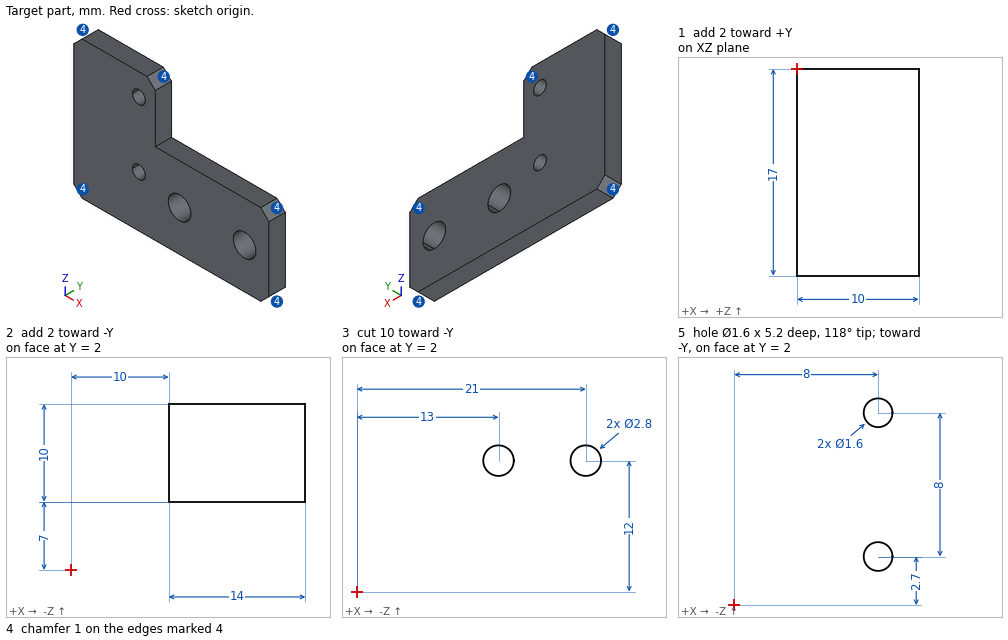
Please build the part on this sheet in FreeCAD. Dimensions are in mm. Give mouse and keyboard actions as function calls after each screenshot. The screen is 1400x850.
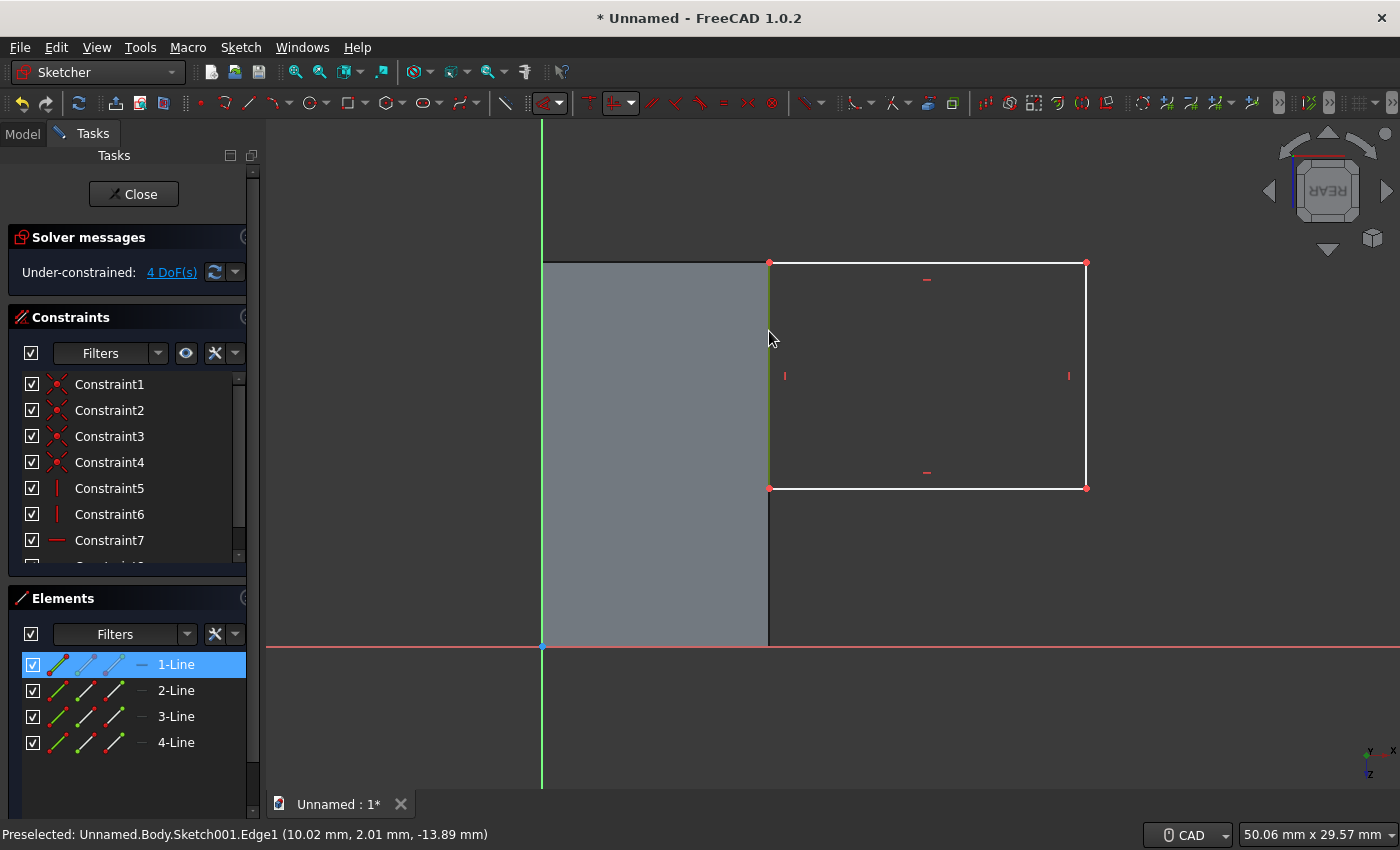
key(i)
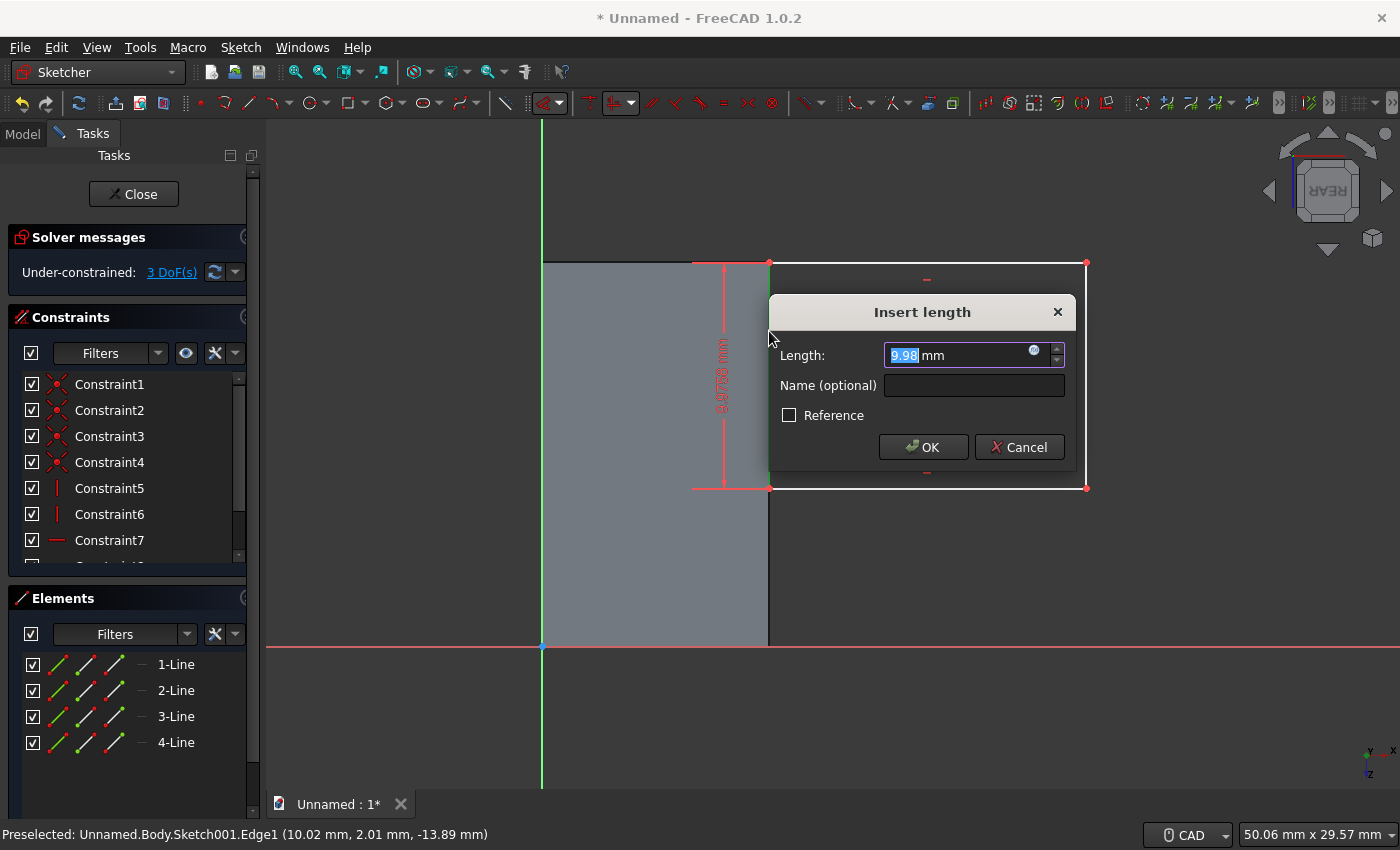
text(10)
key(Return)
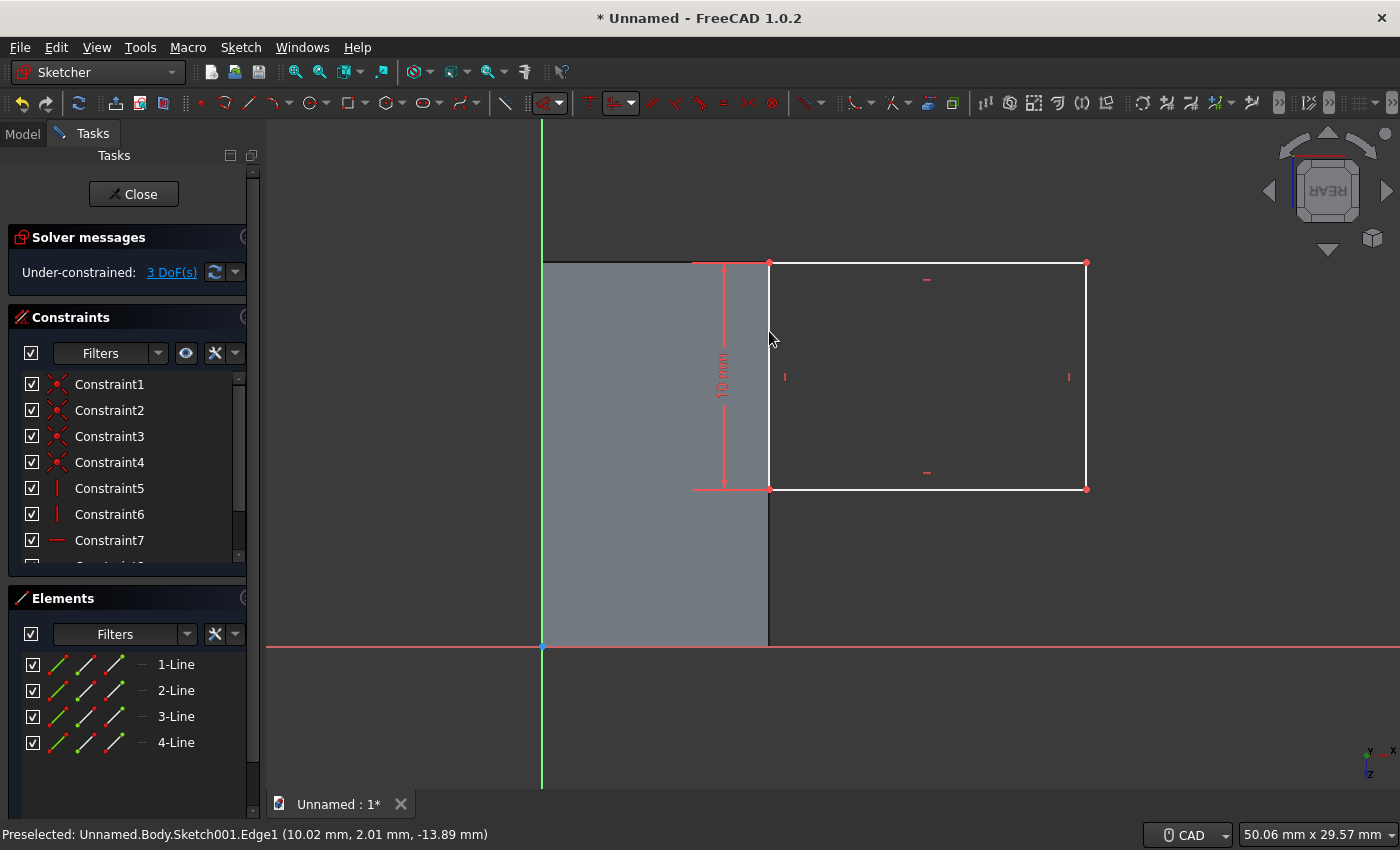
click(864, 490)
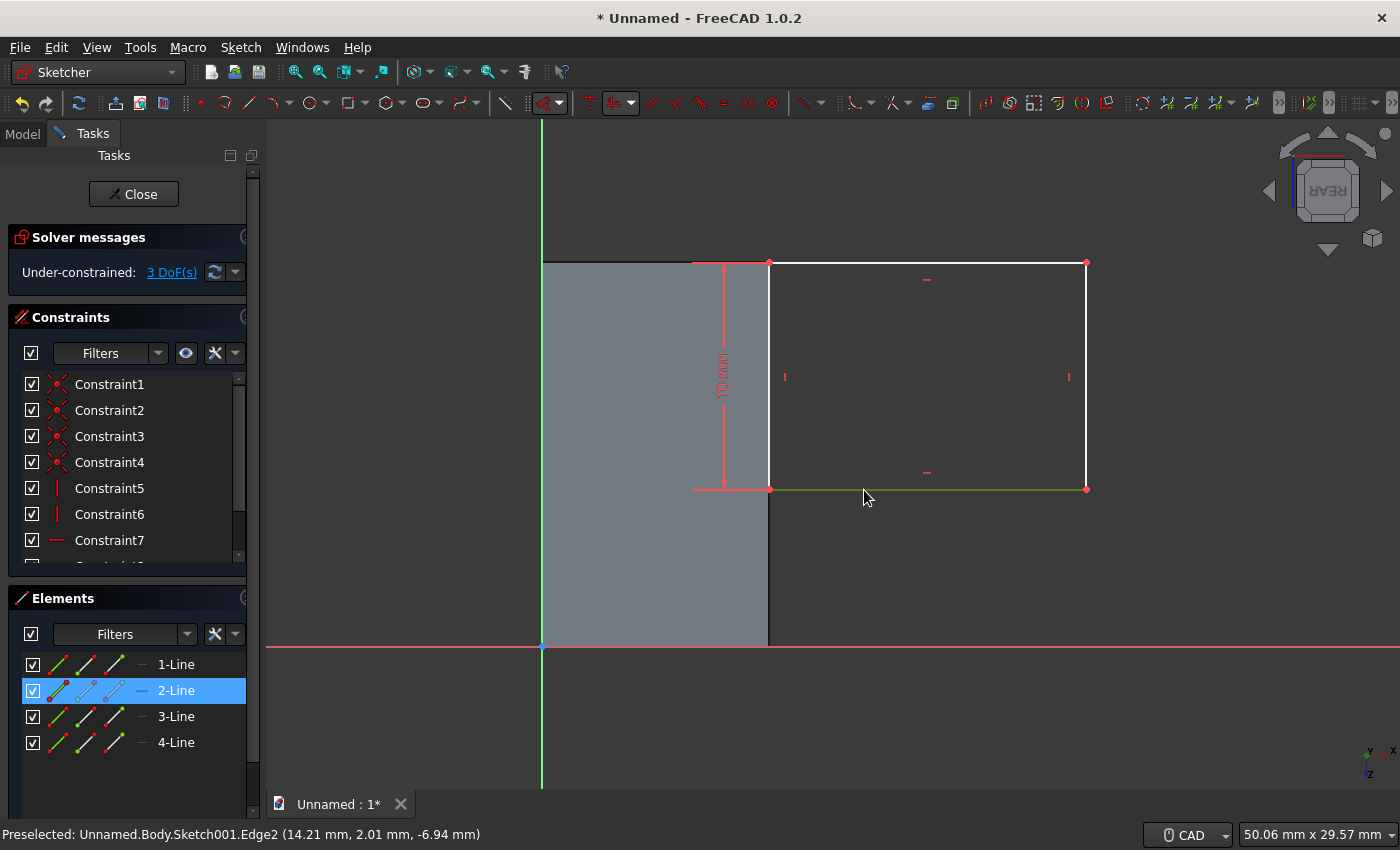
click(562, 104)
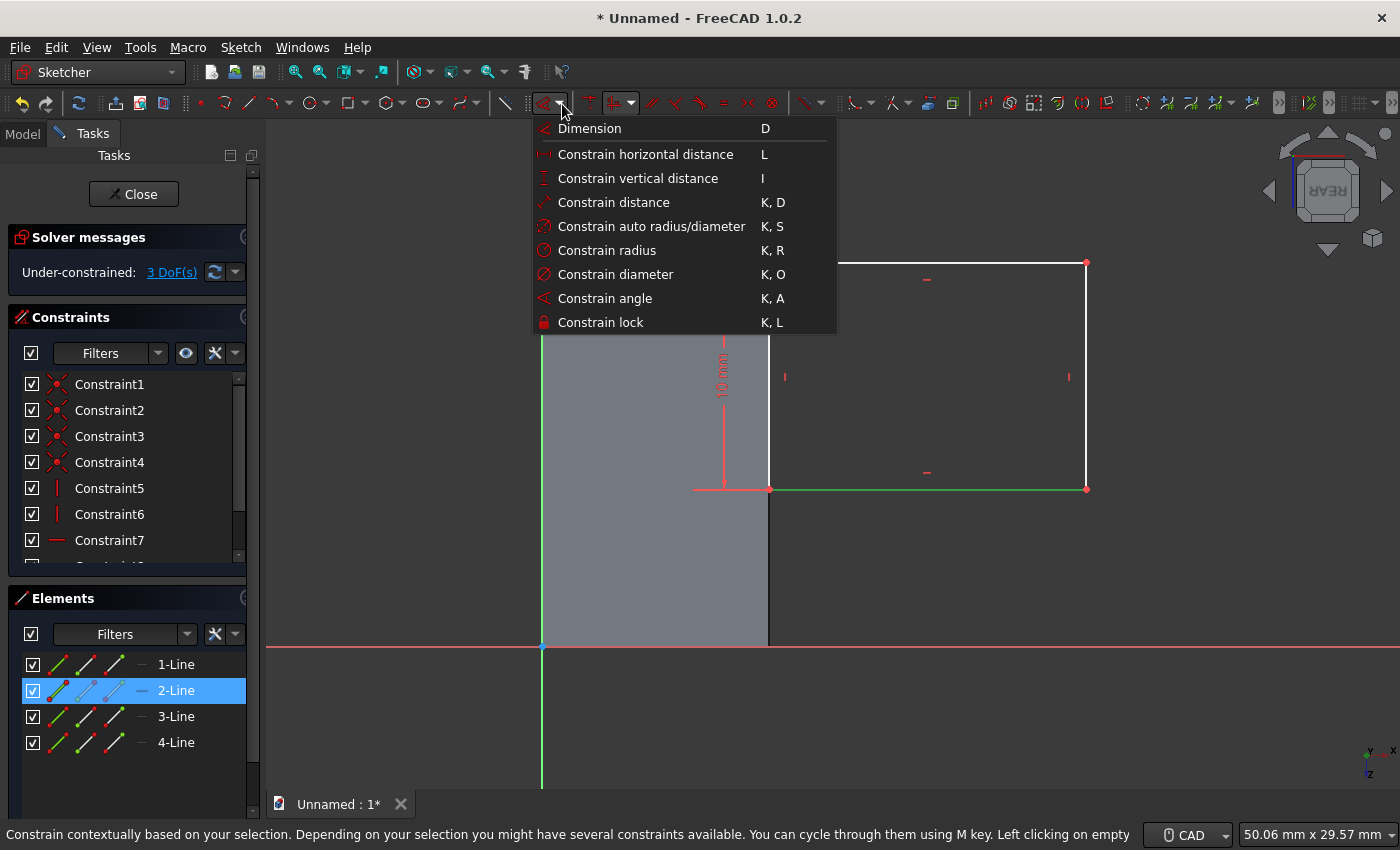
click(685, 154)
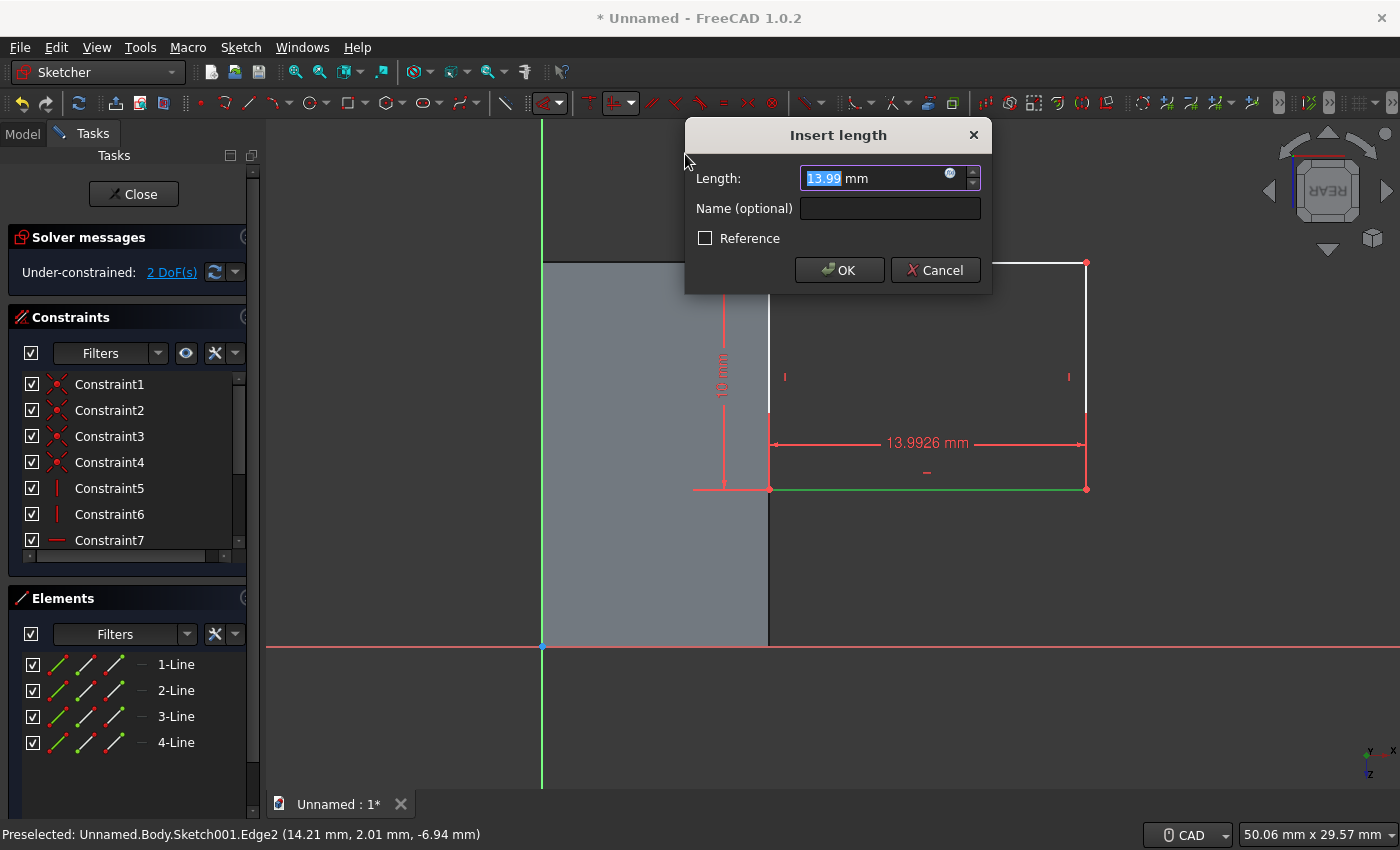
text(14)
key(Return)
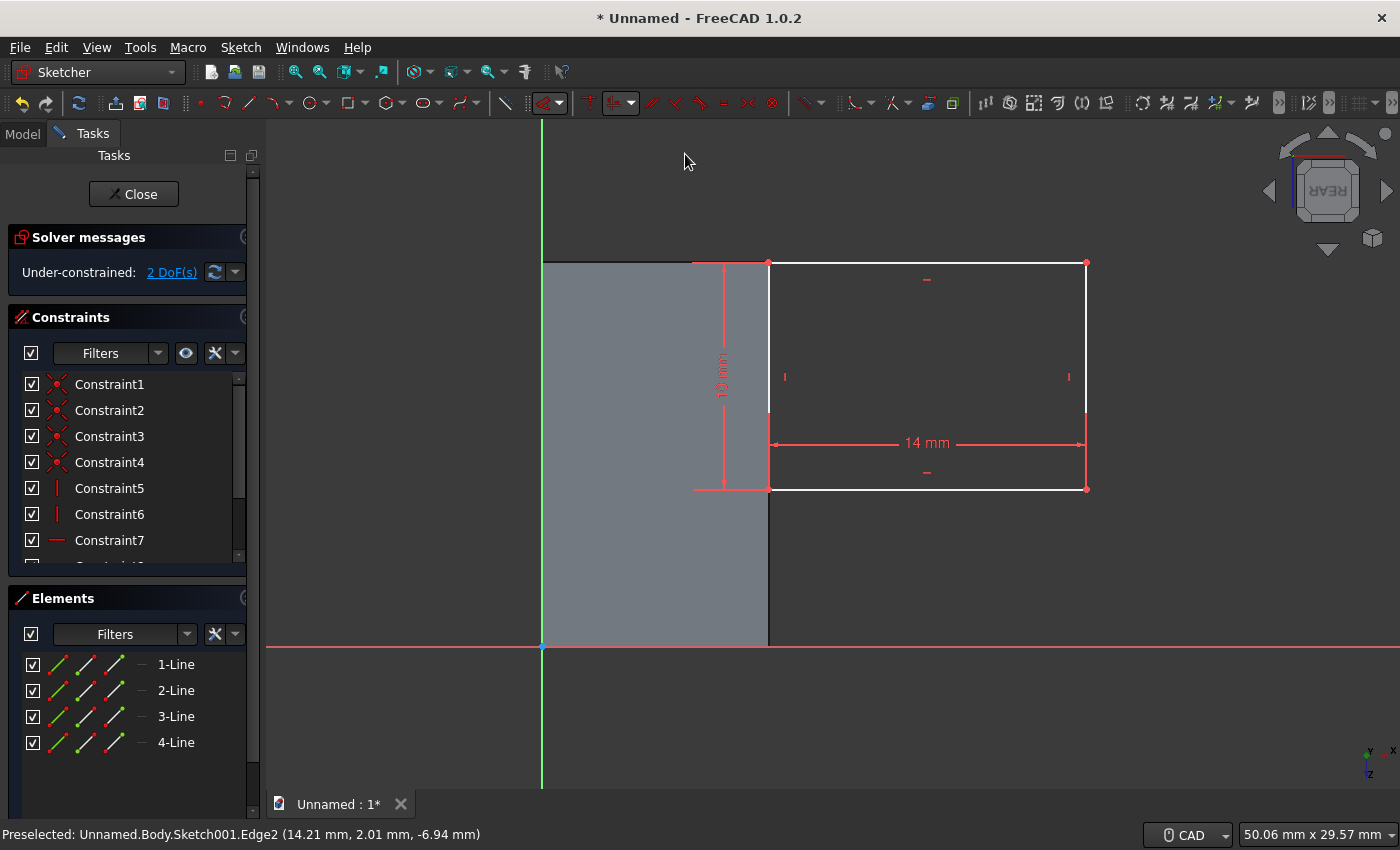
click(769, 490)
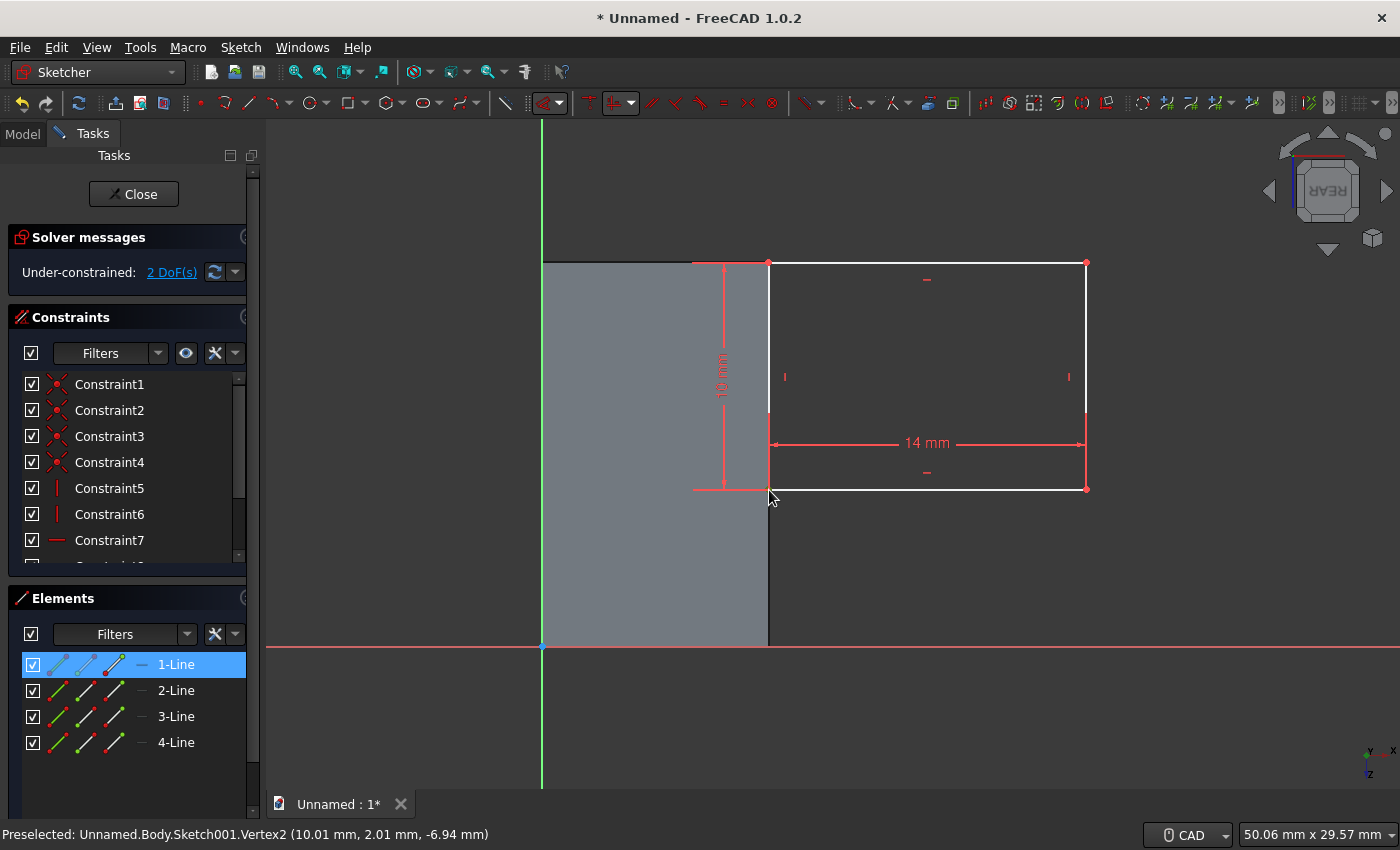
click(562, 104)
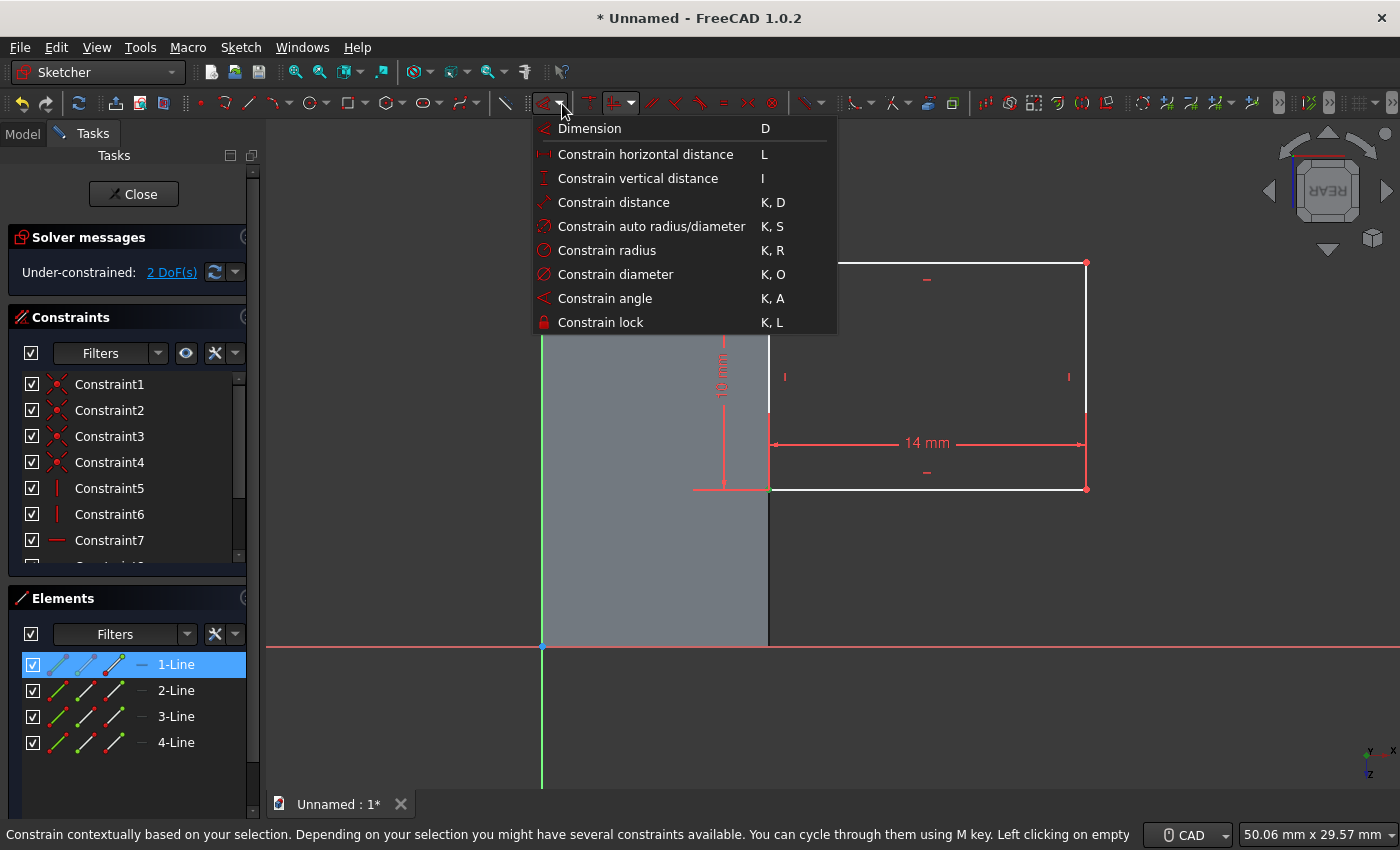
click(685, 178)